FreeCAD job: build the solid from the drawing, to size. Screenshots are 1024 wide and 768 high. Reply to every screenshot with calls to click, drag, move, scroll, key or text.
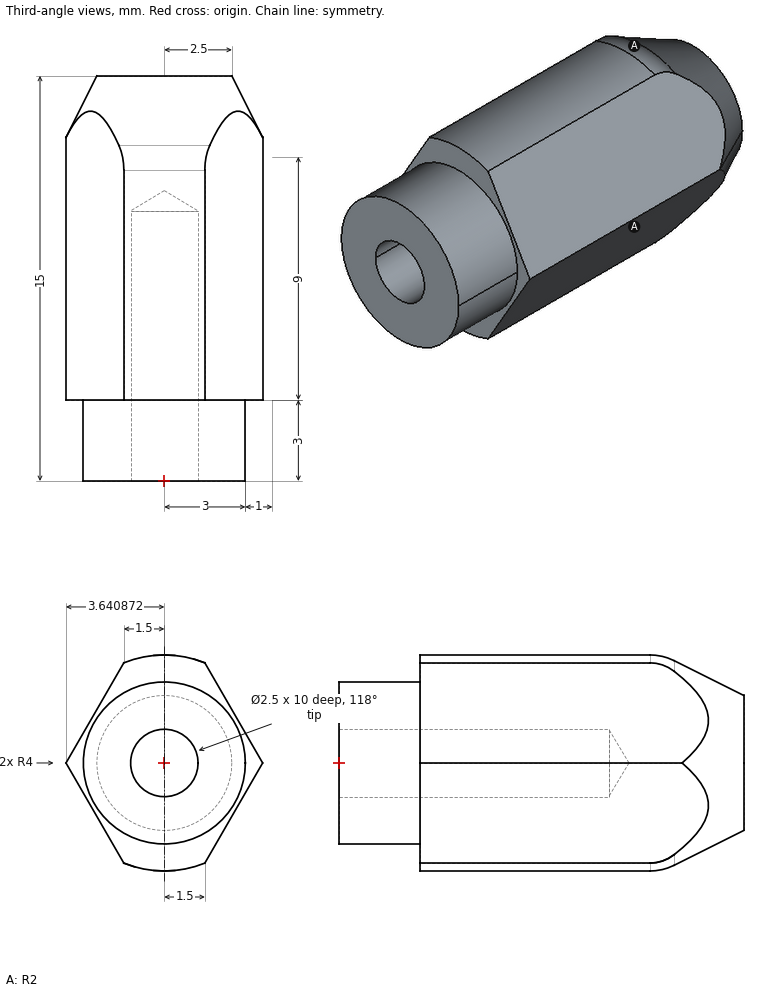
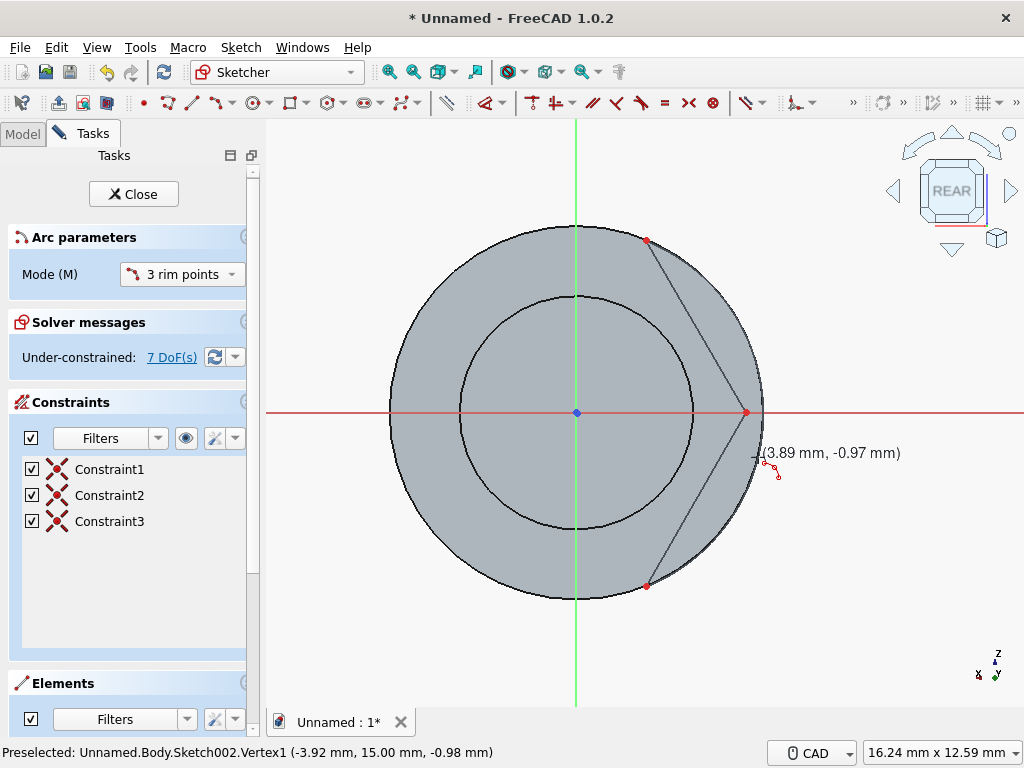
click(168, 104)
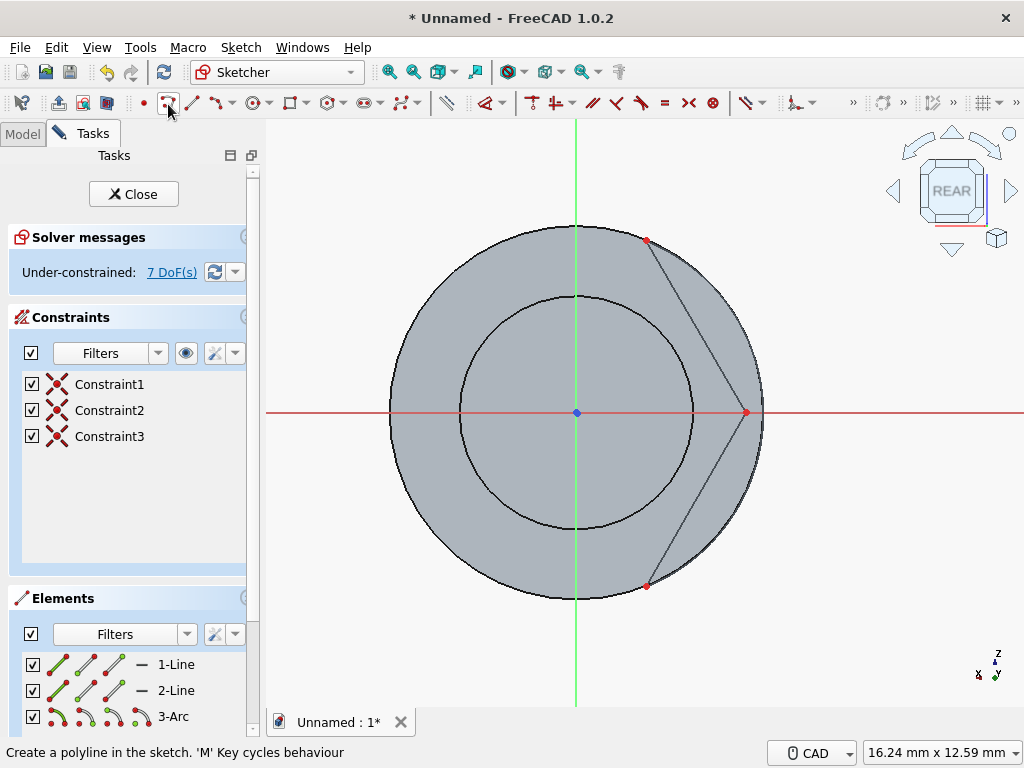
click(506, 586)
click(406, 413)
click(506, 240)
right_click(506, 240)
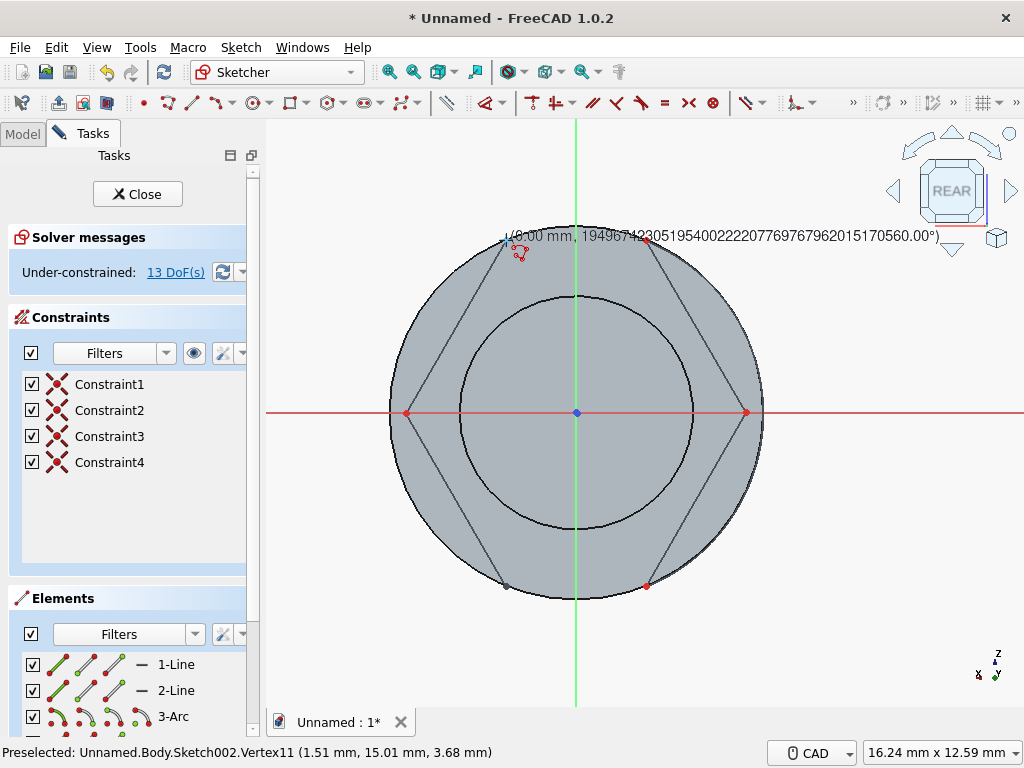
click(216, 104)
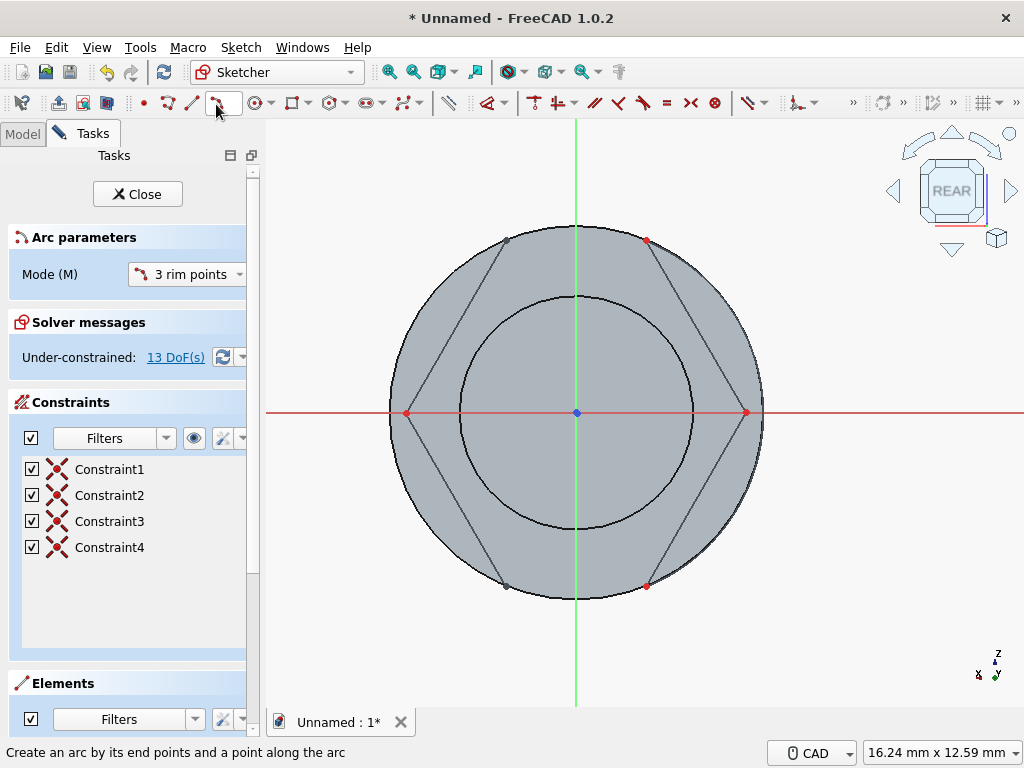
click(506, 241)
click(506, 587)
click(395, 369)
key(Escape)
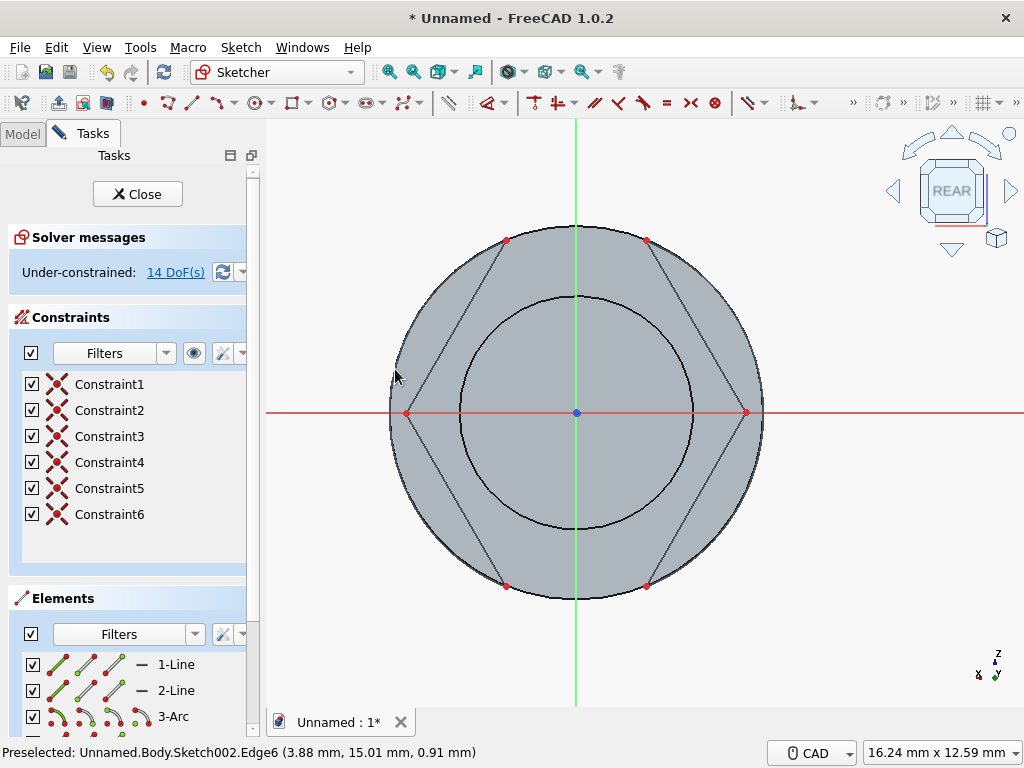
click(743, 499)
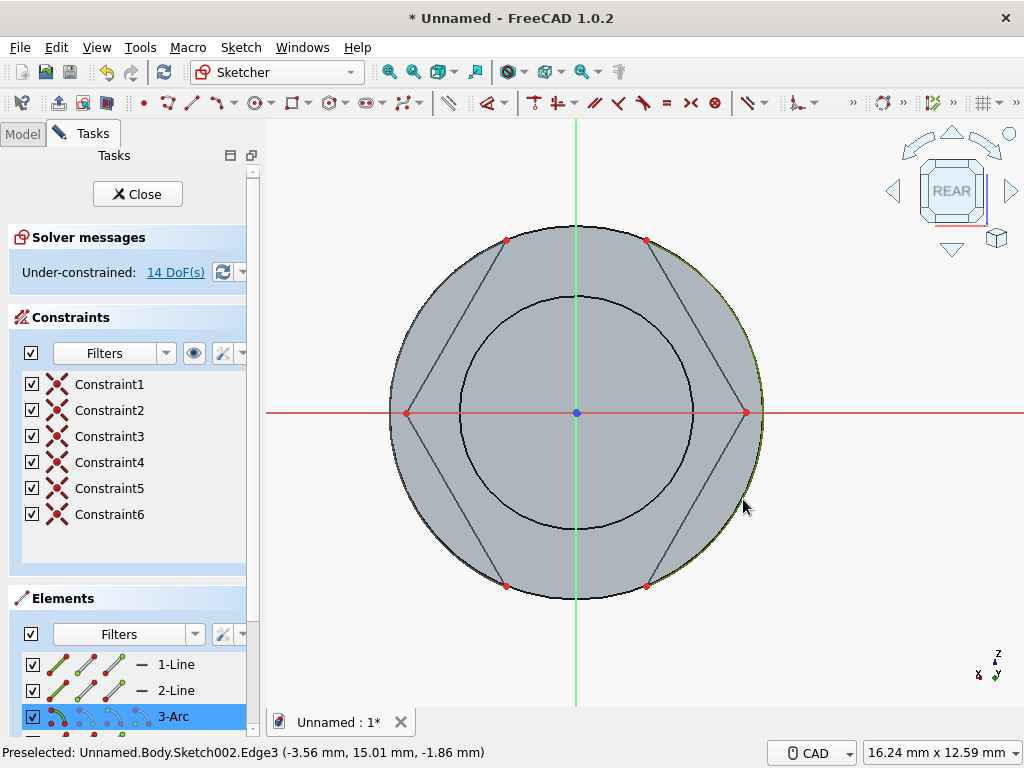
click(410, 329)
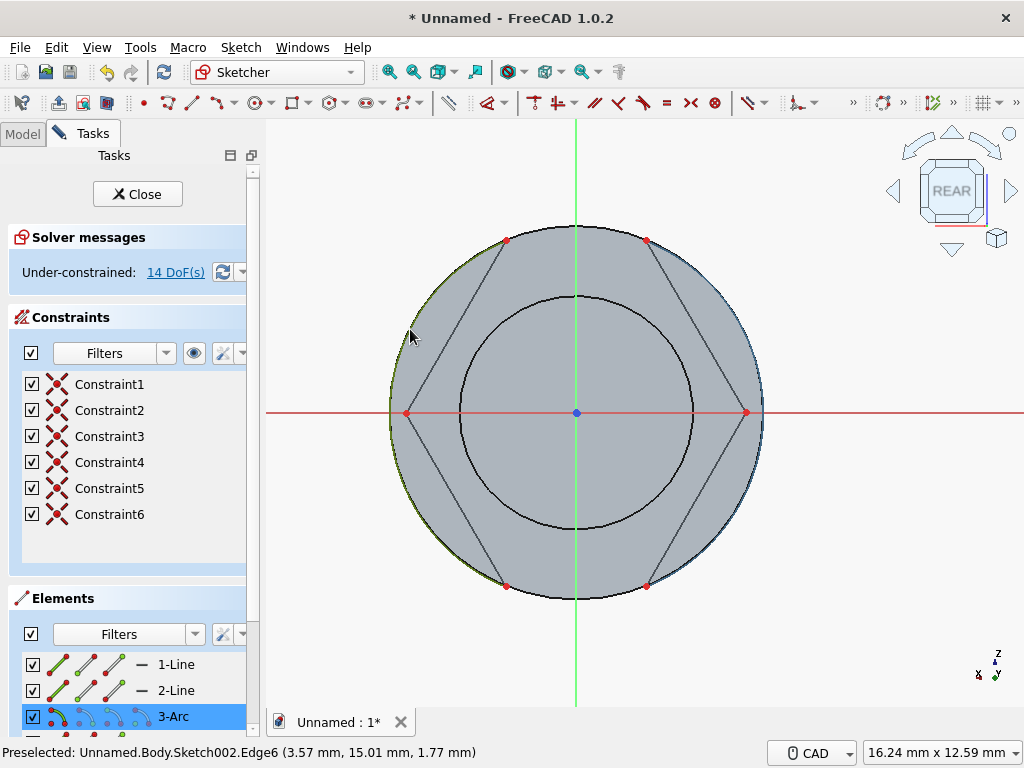
click(534, 104)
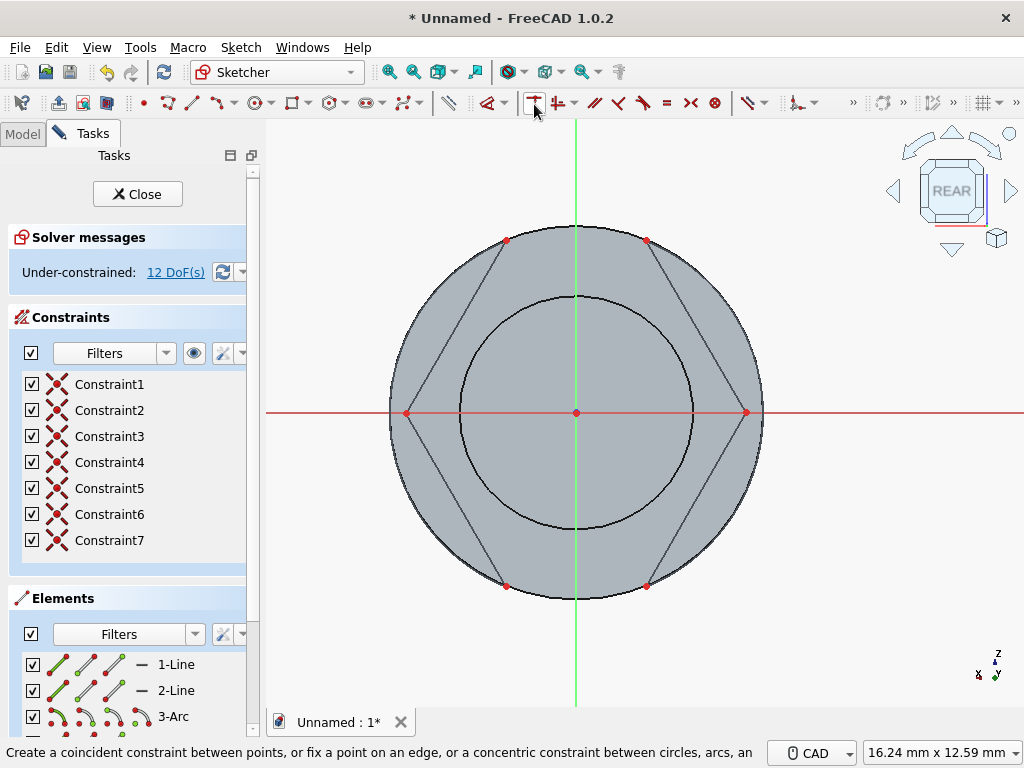
drag(566, 403, 587, 424)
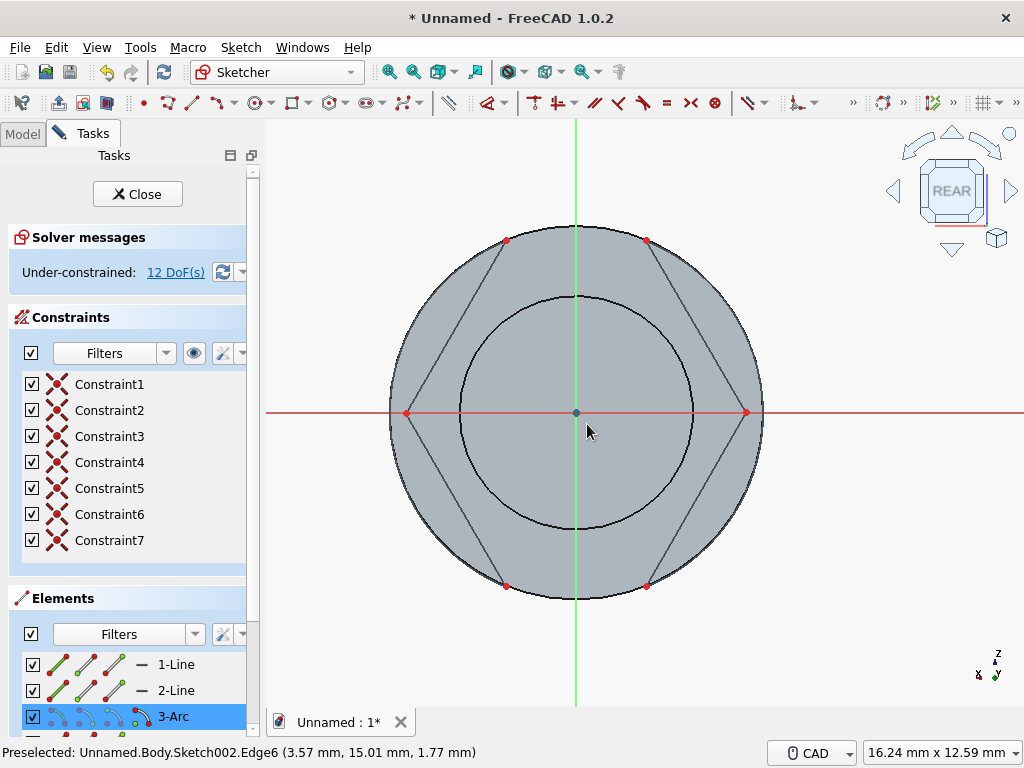
click(534, 104)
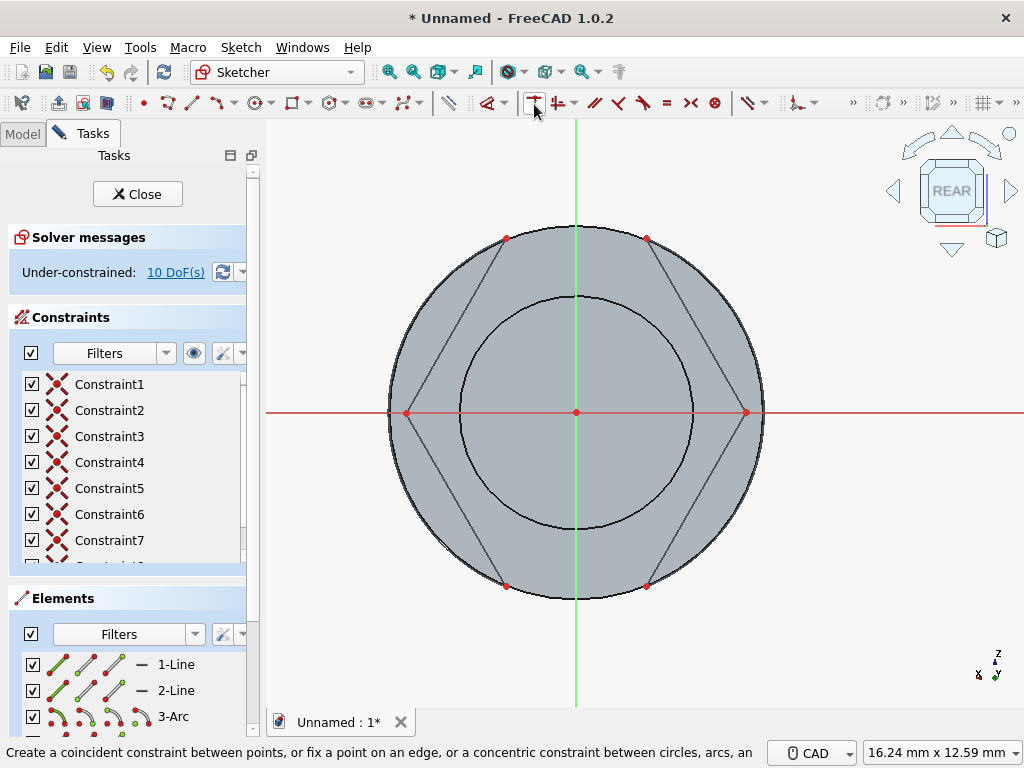
click(743, 499)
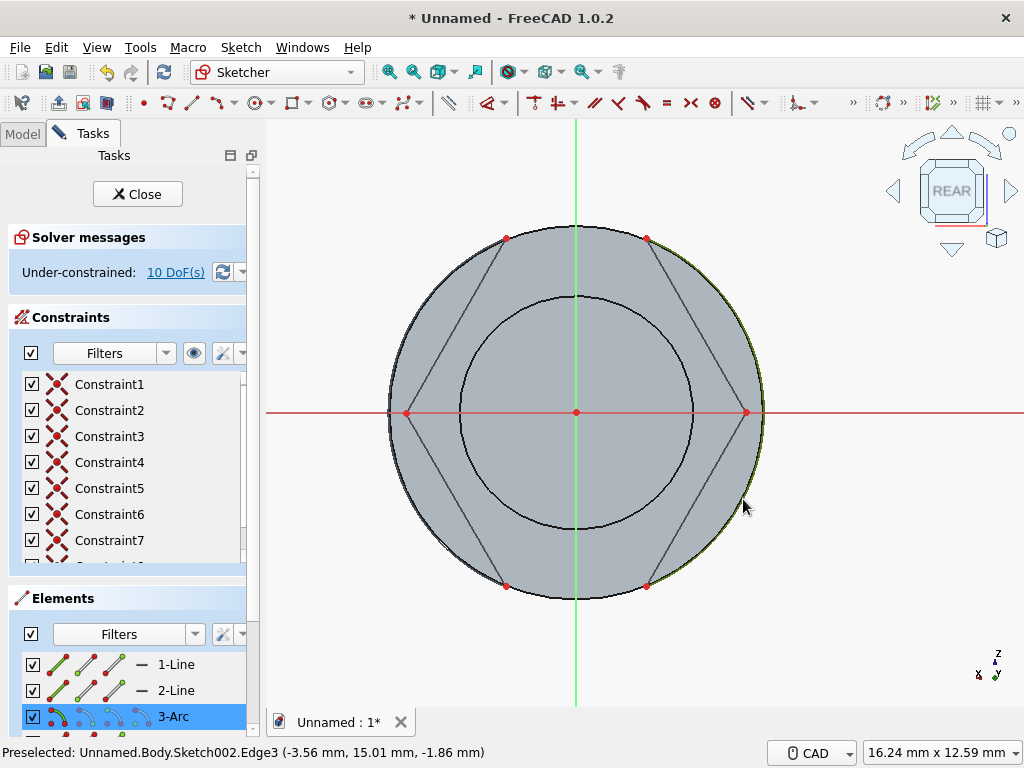
click(409, 327)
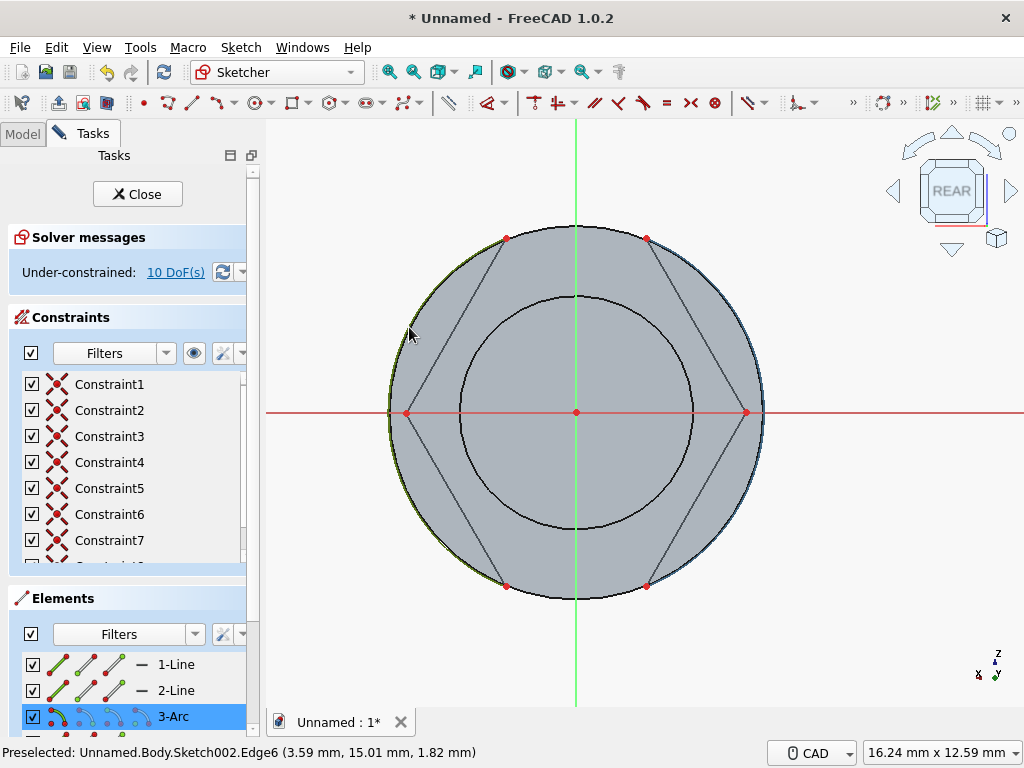
click(668, 104)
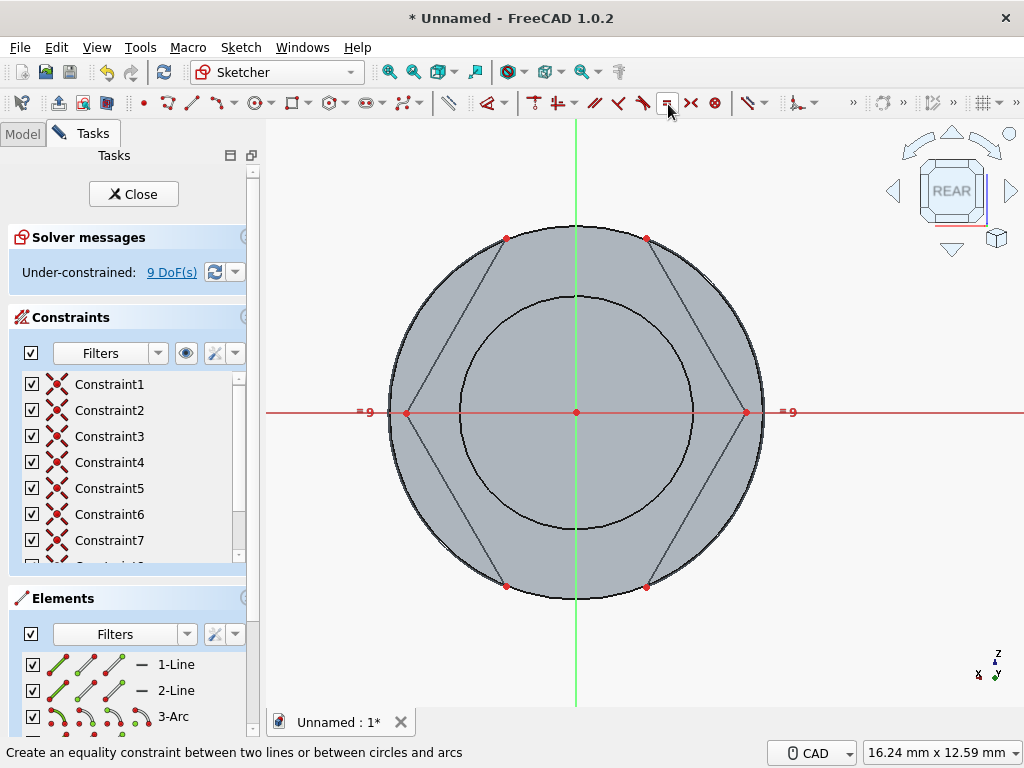
click(746, 413)